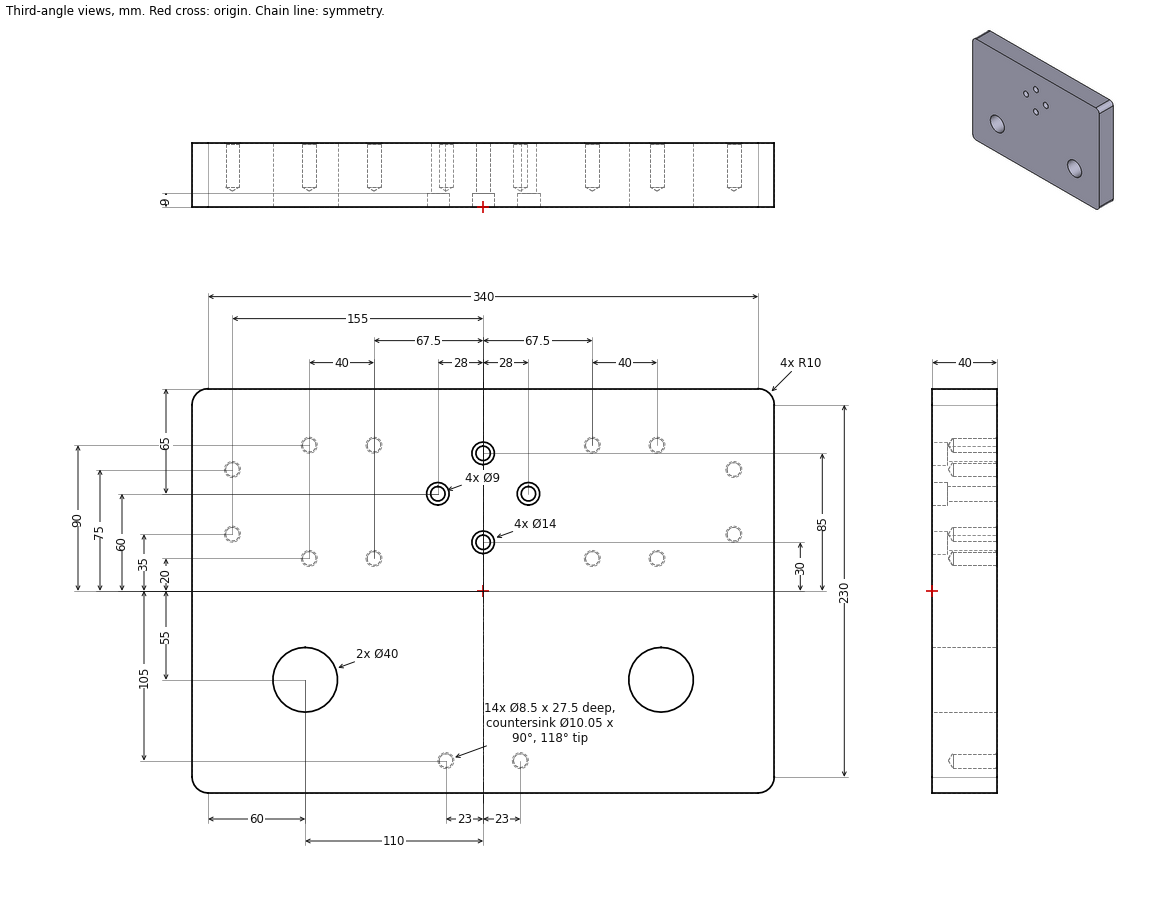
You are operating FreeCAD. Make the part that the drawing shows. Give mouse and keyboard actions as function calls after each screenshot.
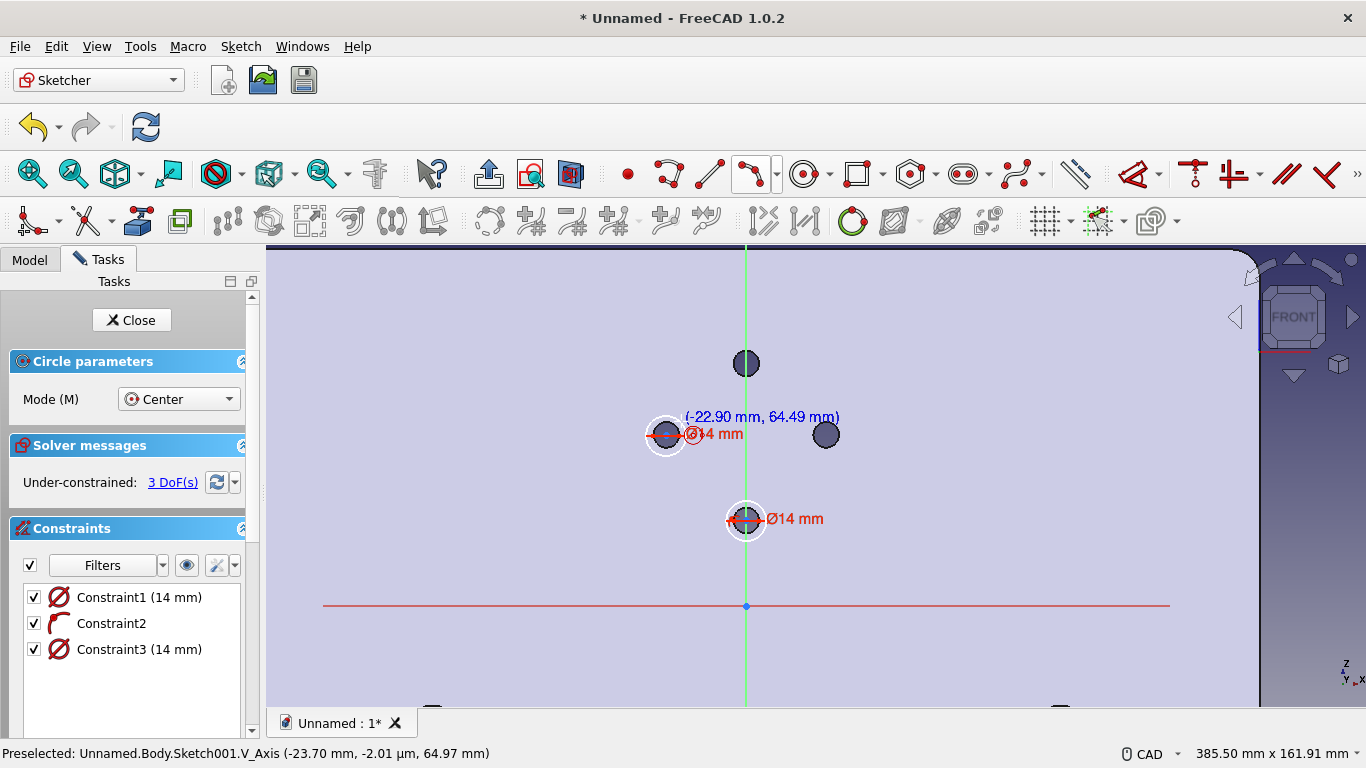
click(746, 363)
move(760, 349)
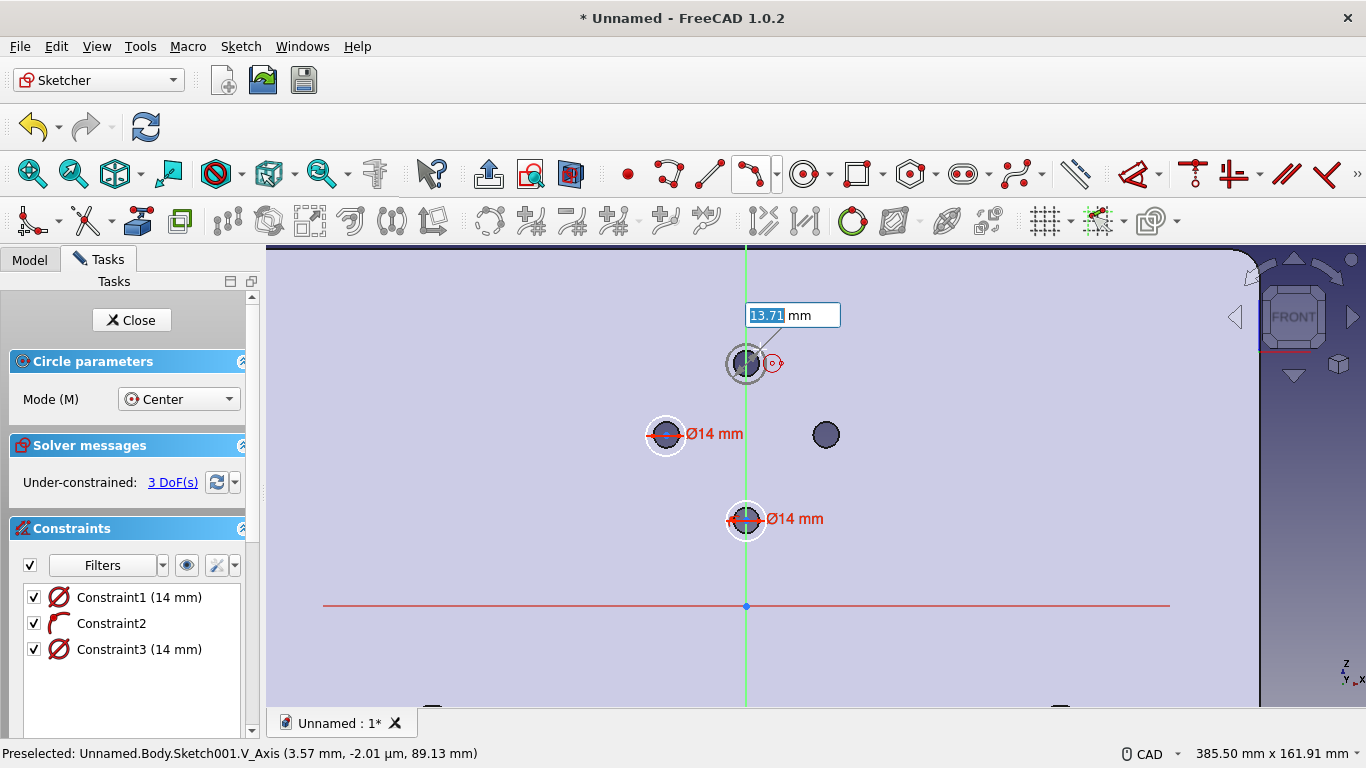
text(14)
key(Return)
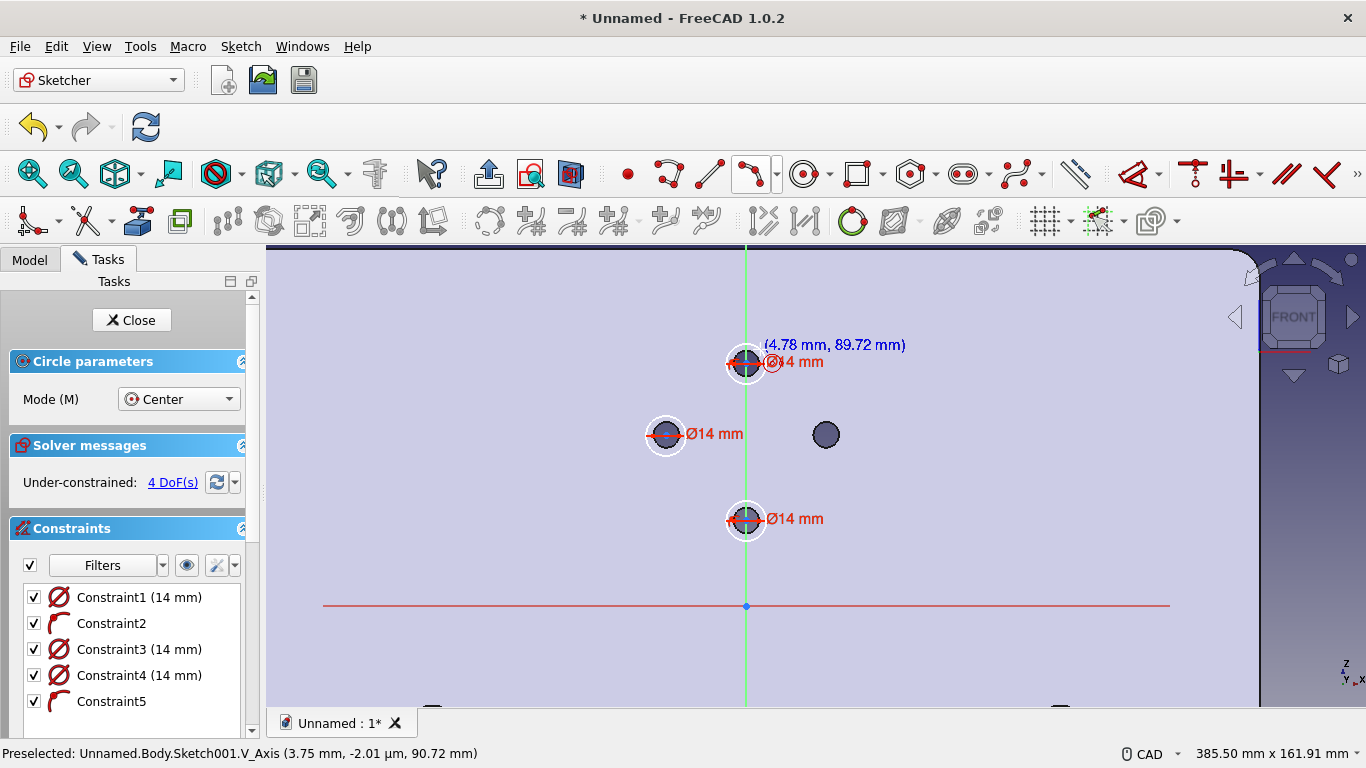
click(826, 435)
move(840, 421)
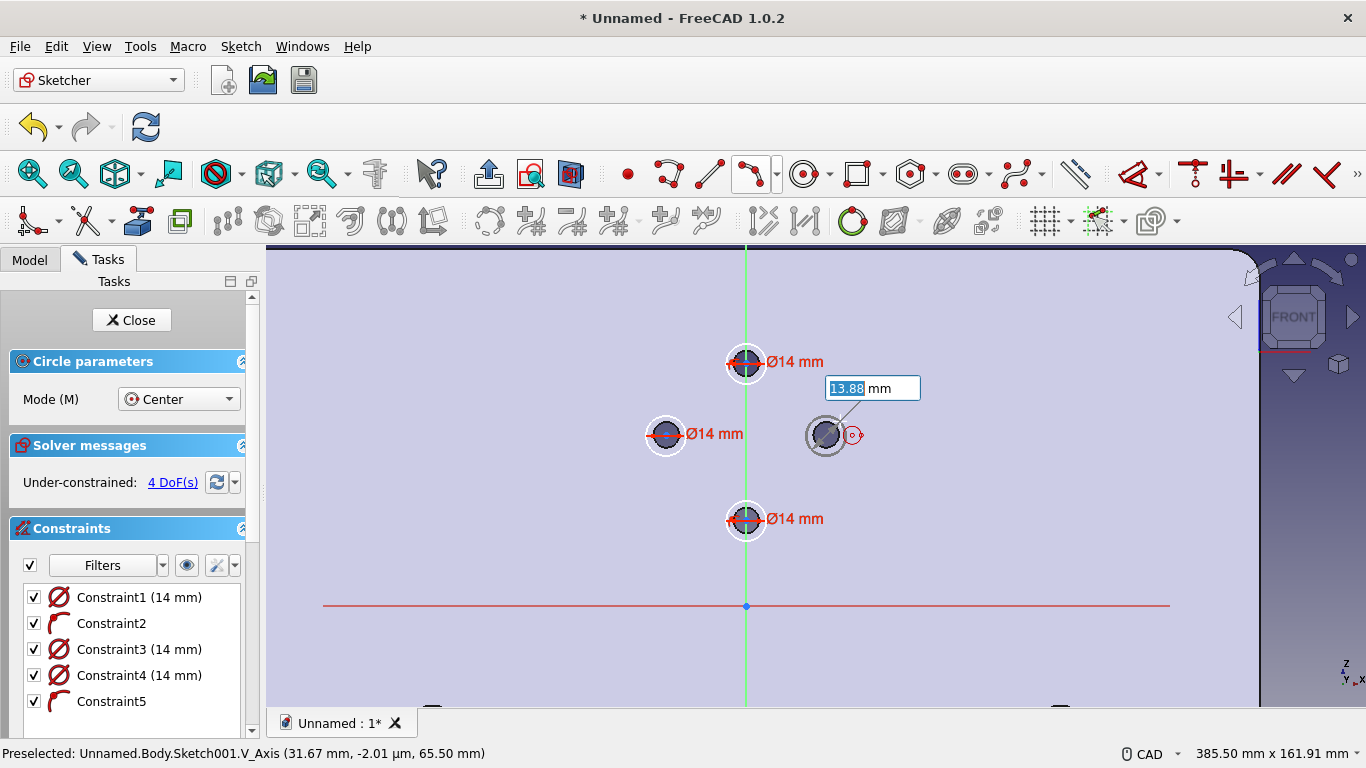
text(14)
key(Return)
key(Escape)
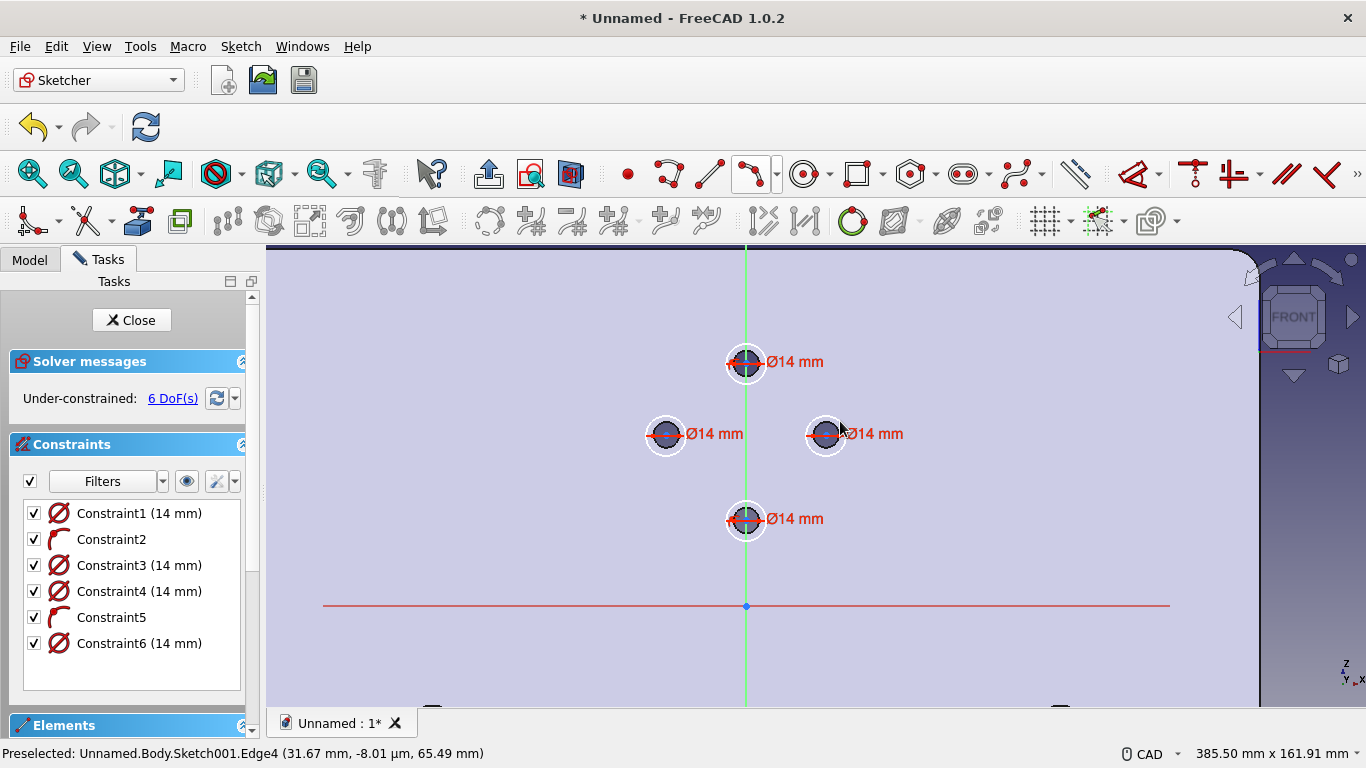
click(666, 436)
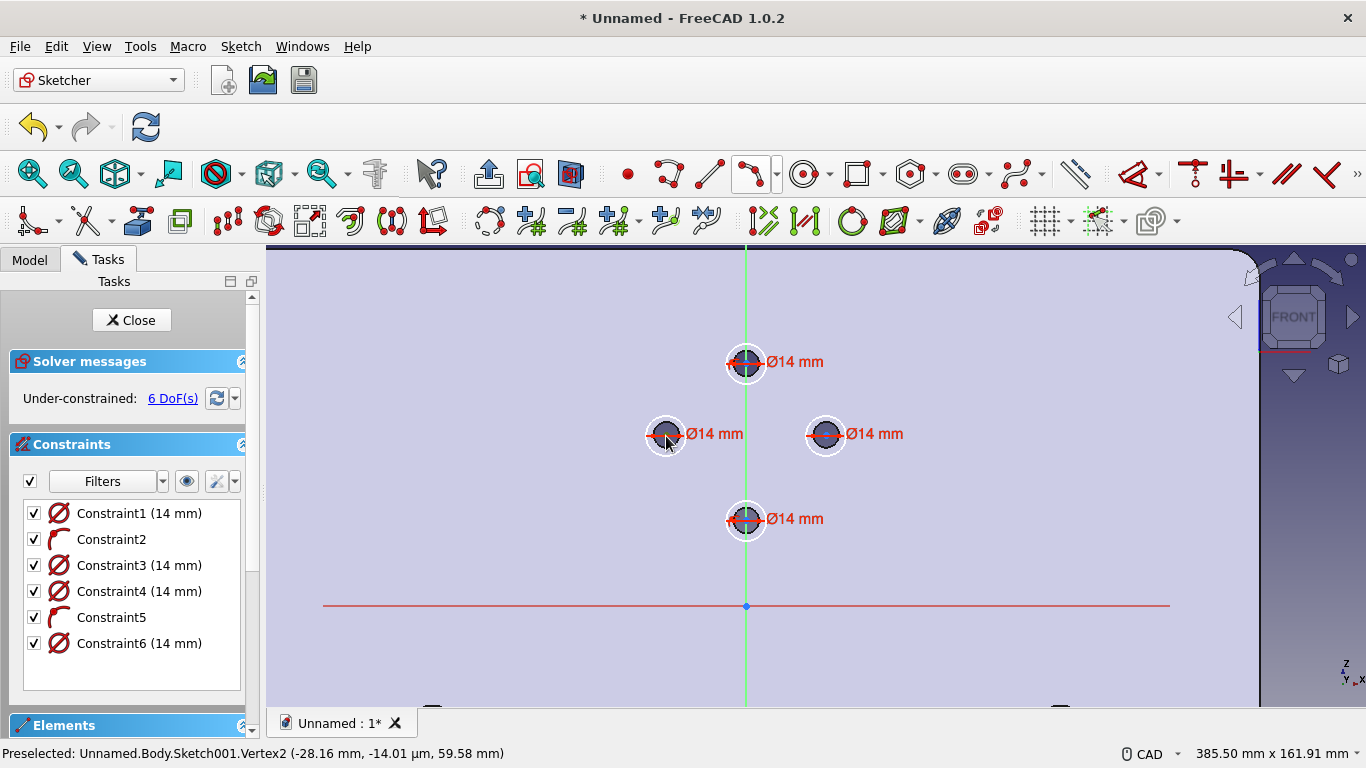
click(826, 436)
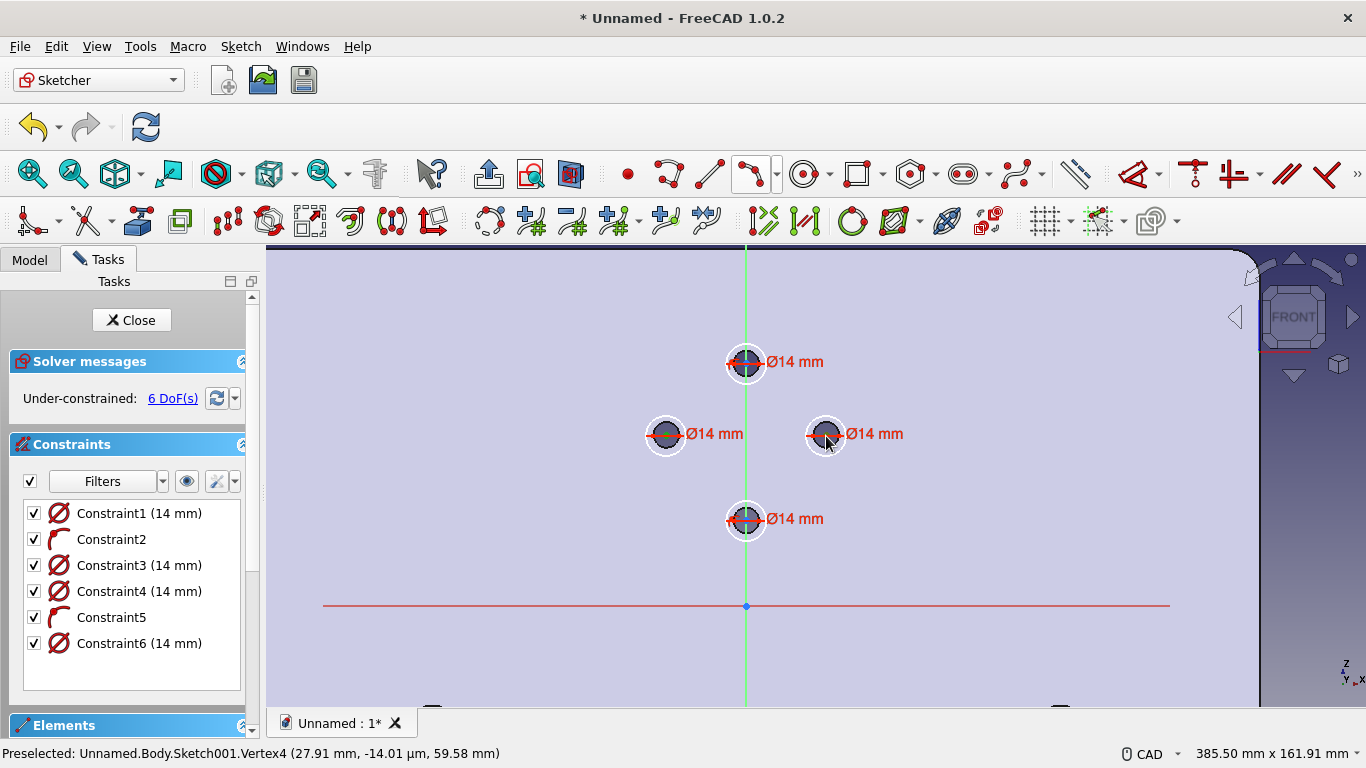
click(1260, 174)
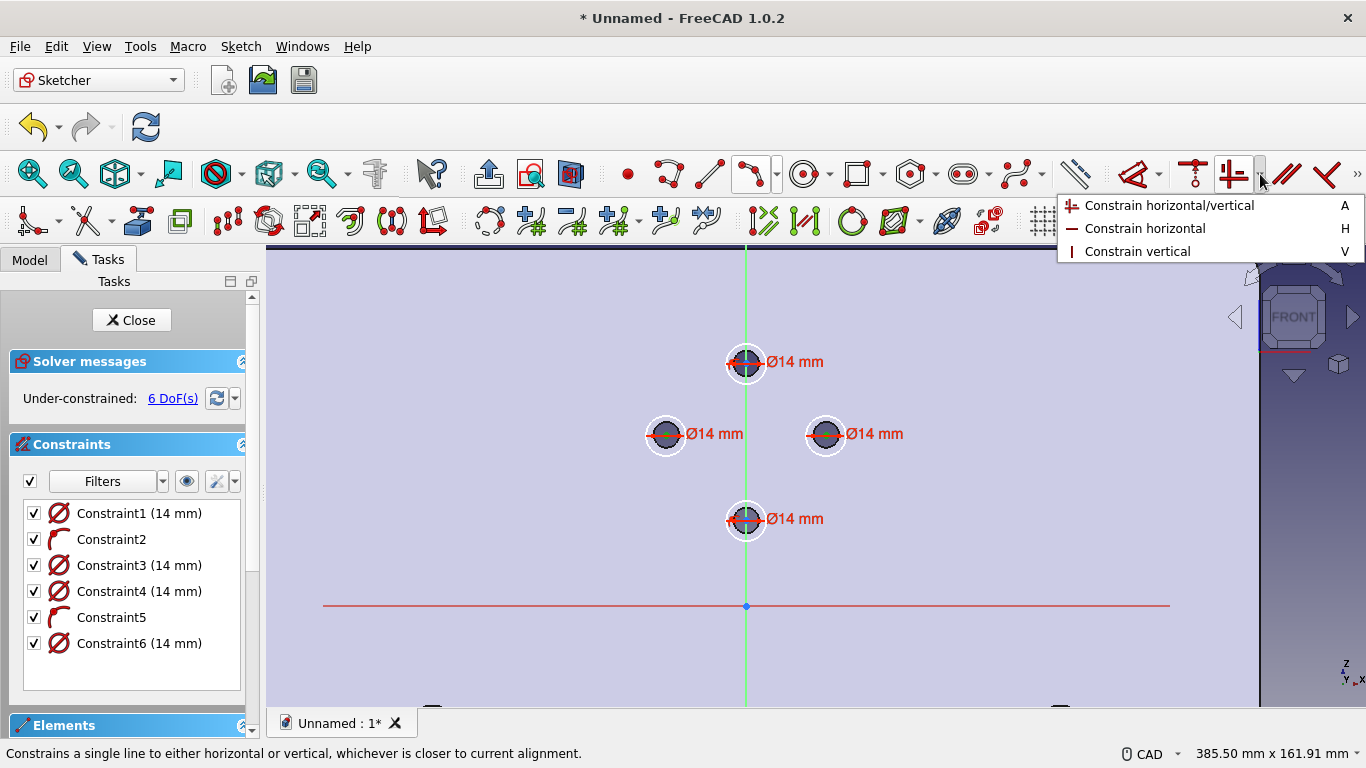
click(1211, 228)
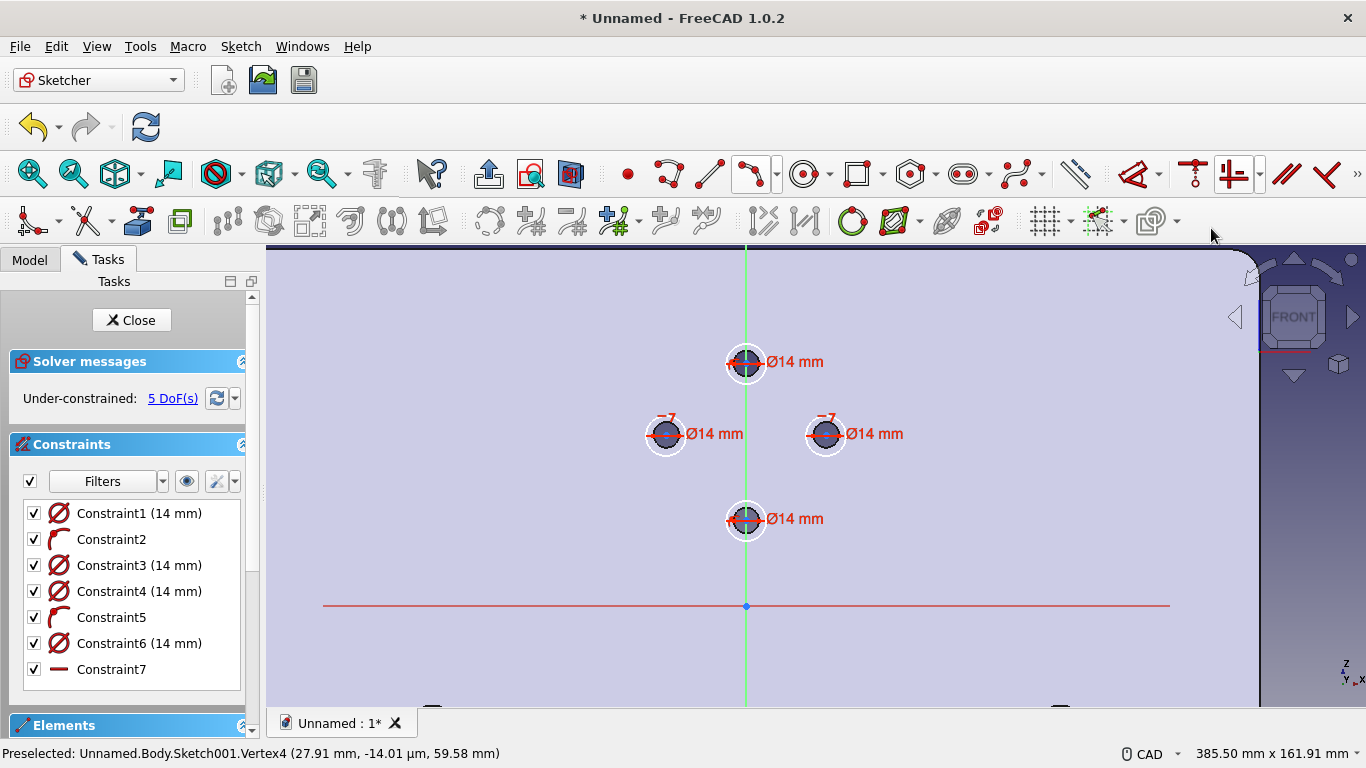
click(1132, 174)